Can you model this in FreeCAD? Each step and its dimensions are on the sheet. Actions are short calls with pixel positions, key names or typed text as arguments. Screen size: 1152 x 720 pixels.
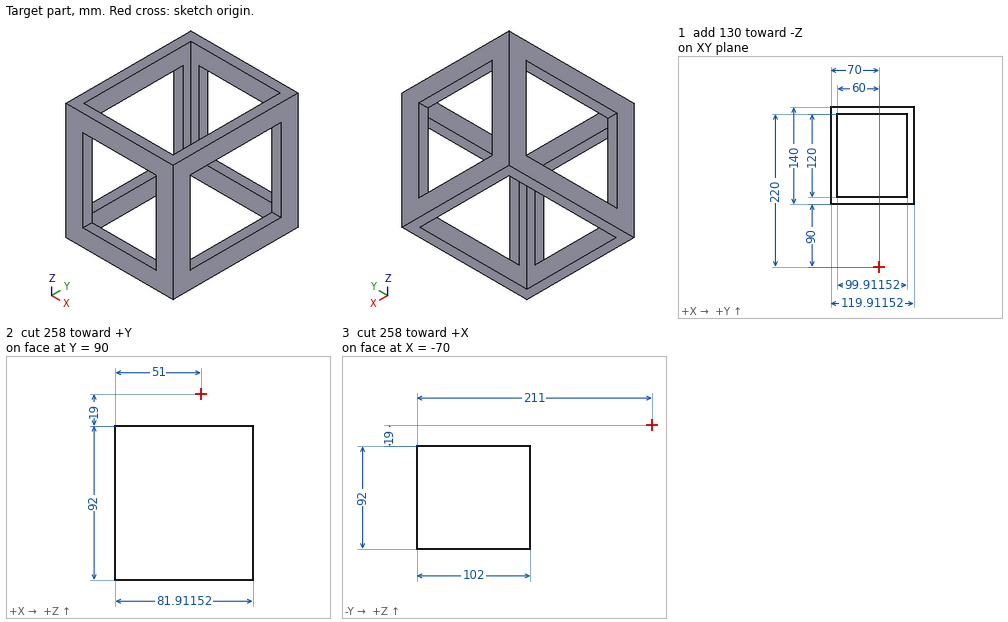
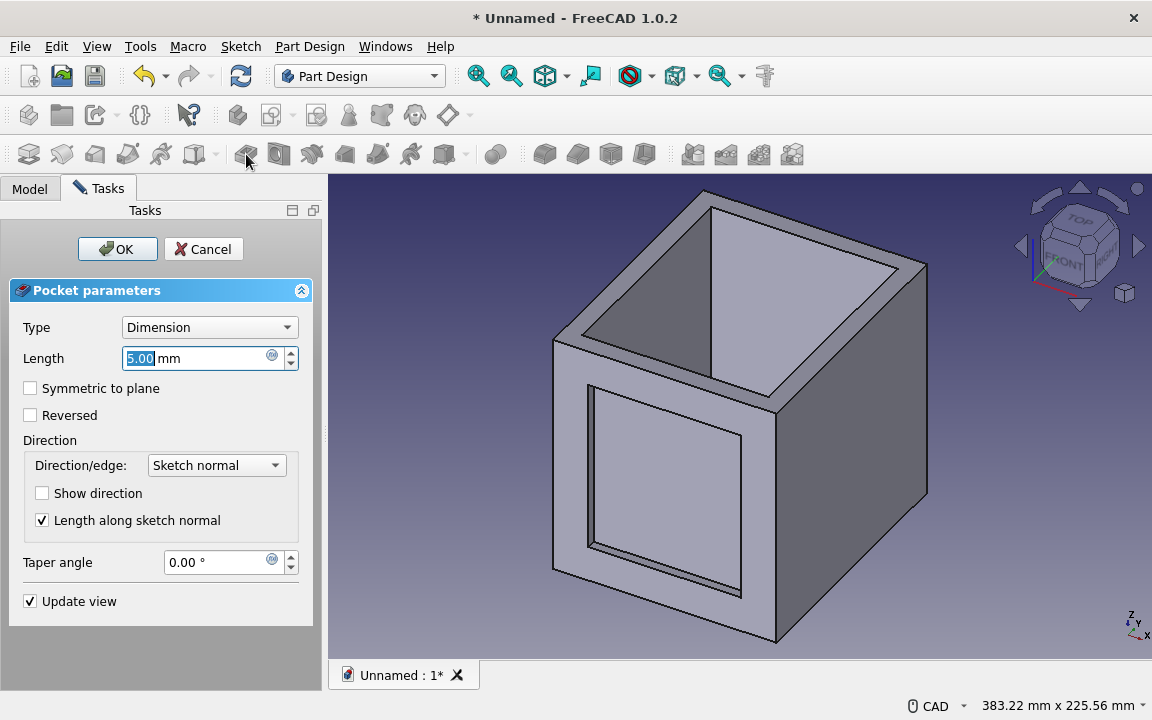
text(258)
key(Tab)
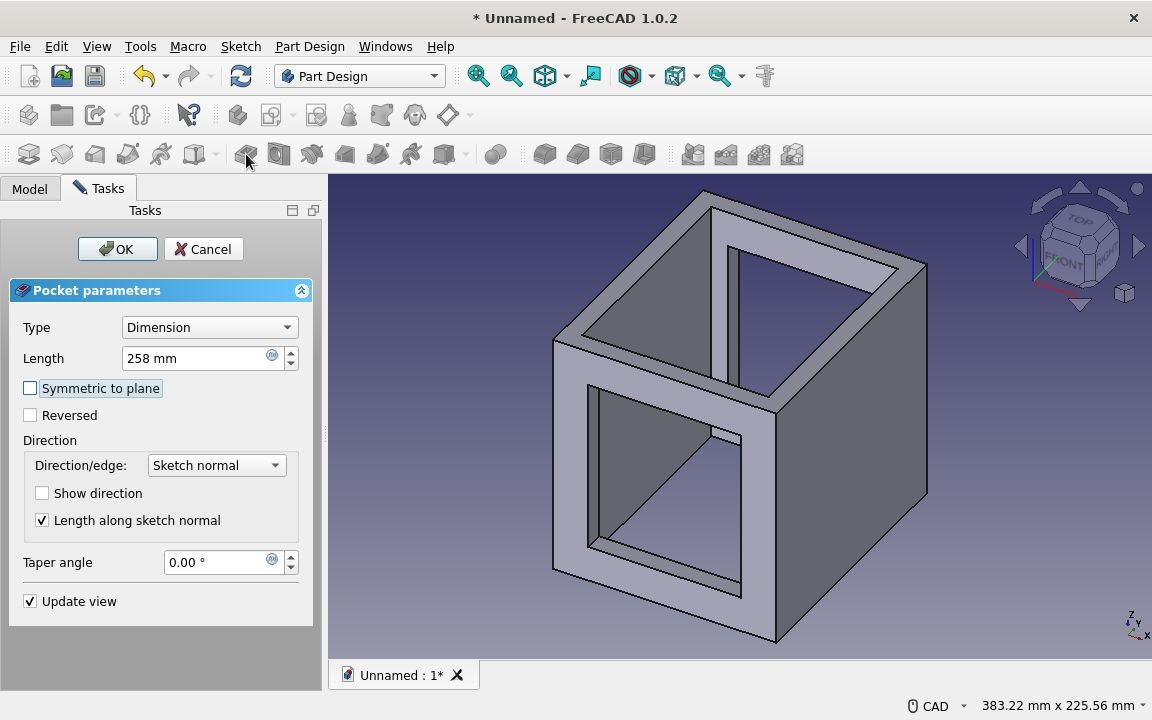
click(118, 249)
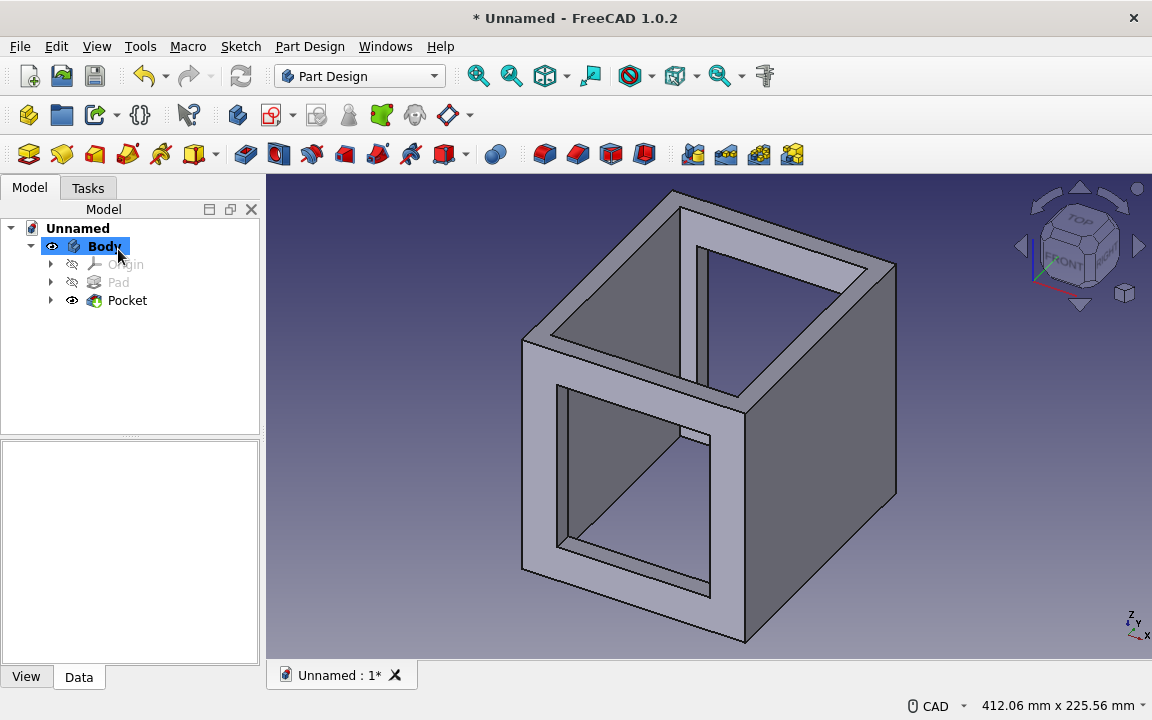
key(6)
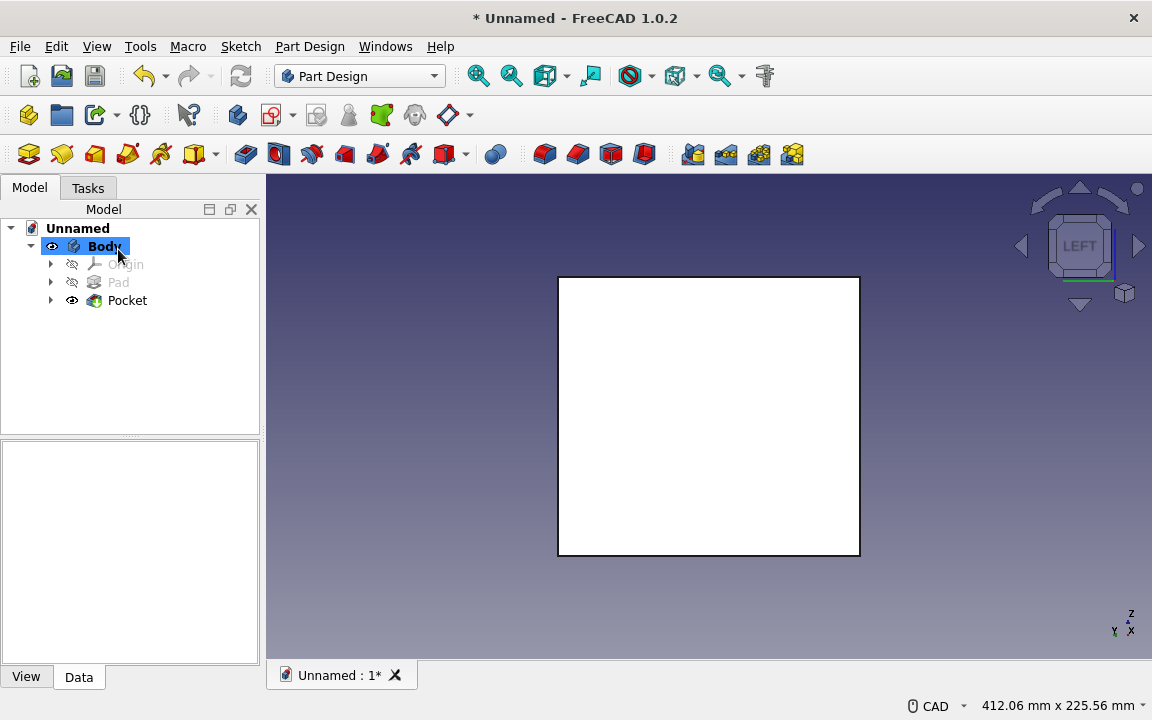
click(709, 415)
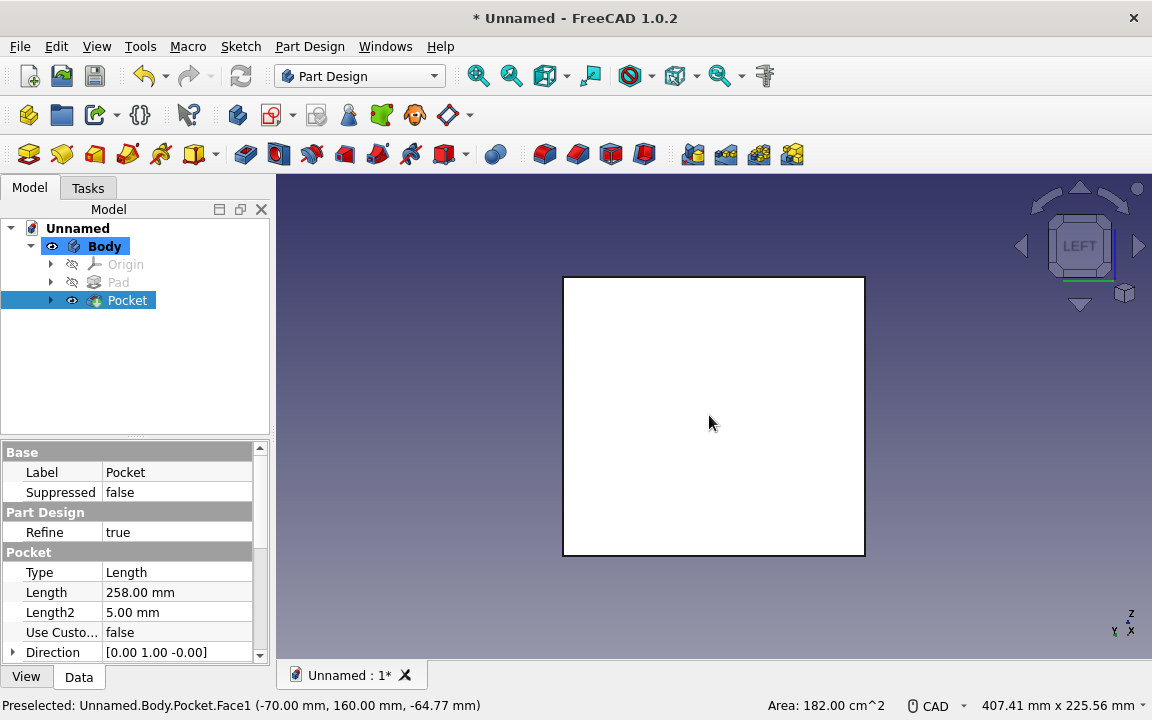
click(270, 116)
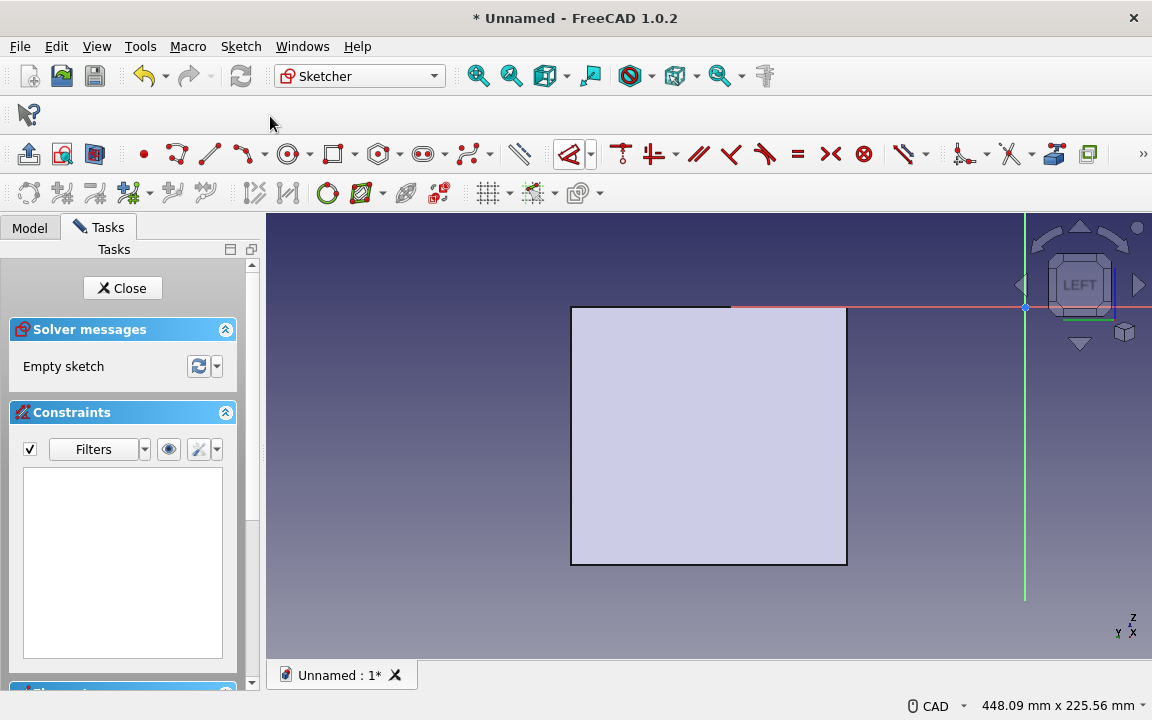
scroll(294, 521, down, 1)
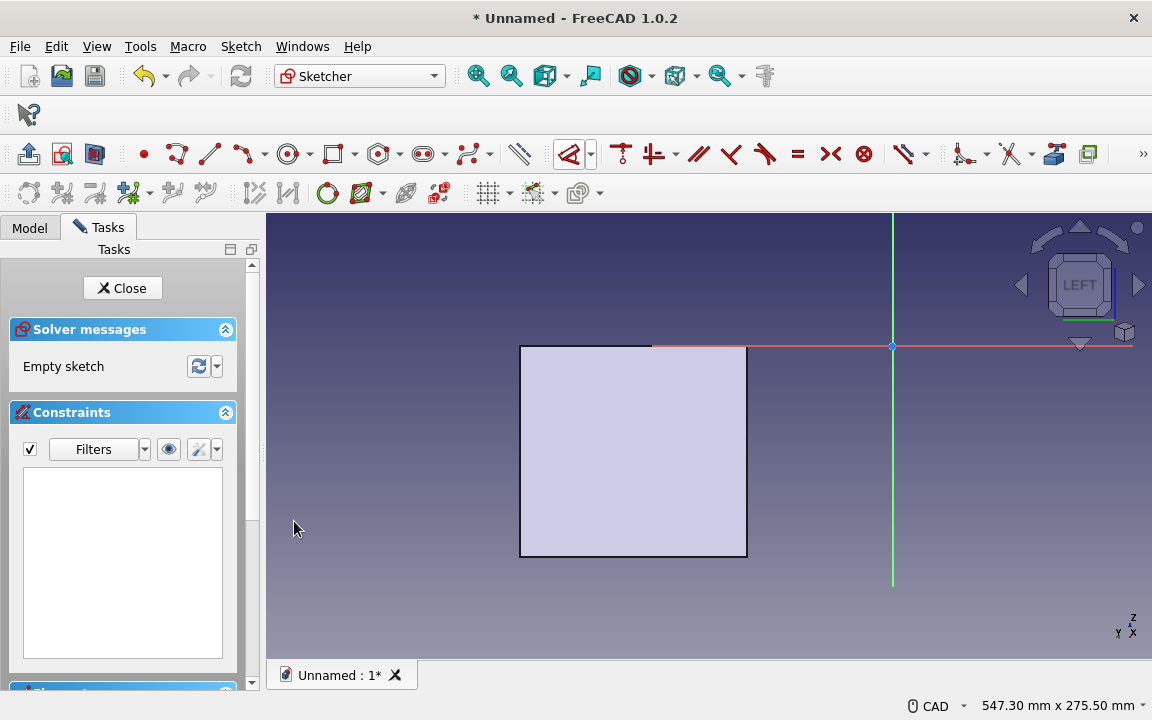
scroll(888, 436, up, 2)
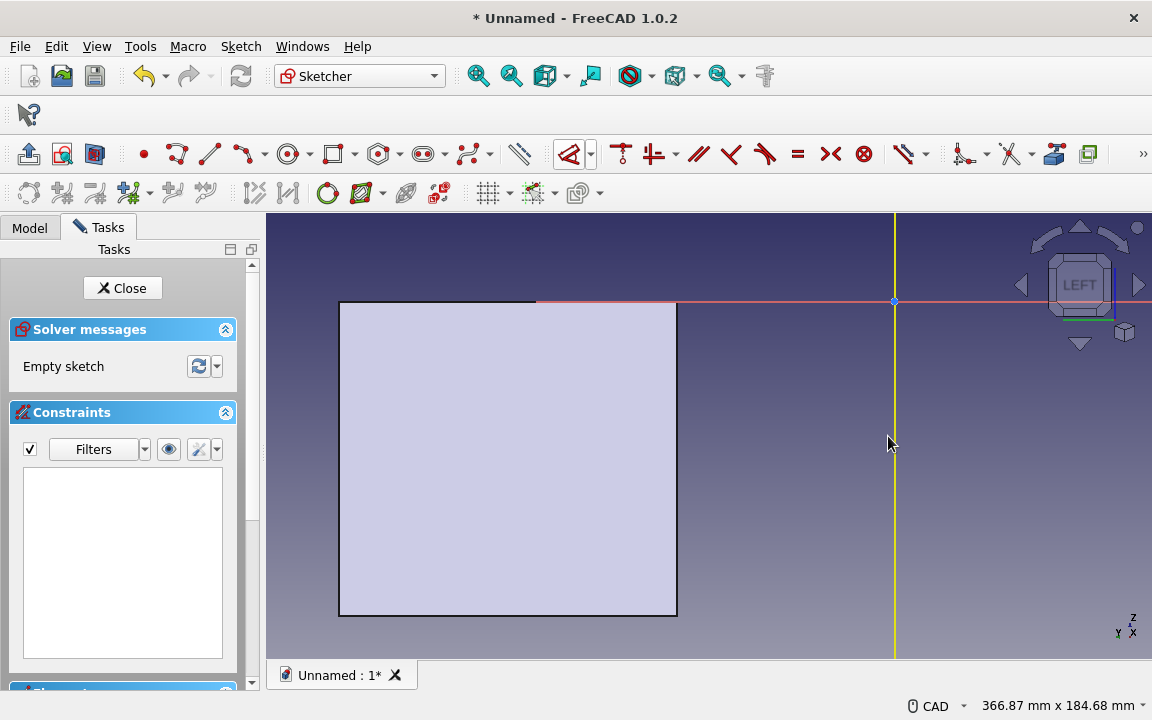
click(332, 154)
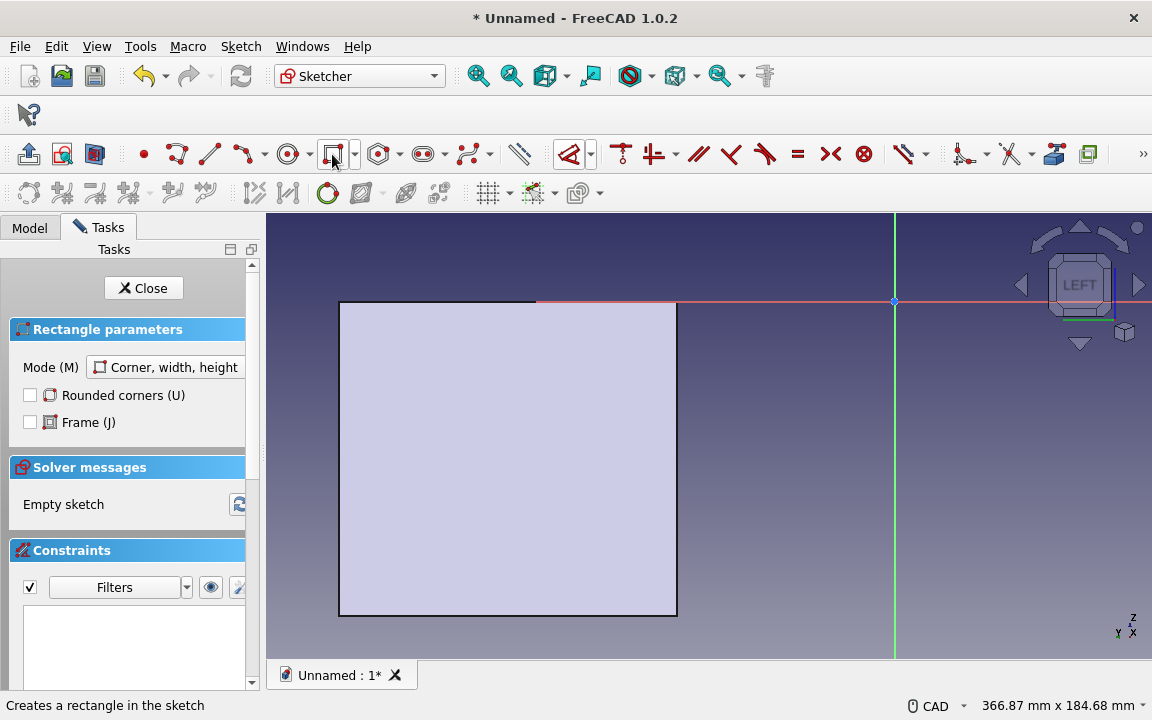
click(385, 348)
click(632, 570)
key(Escape)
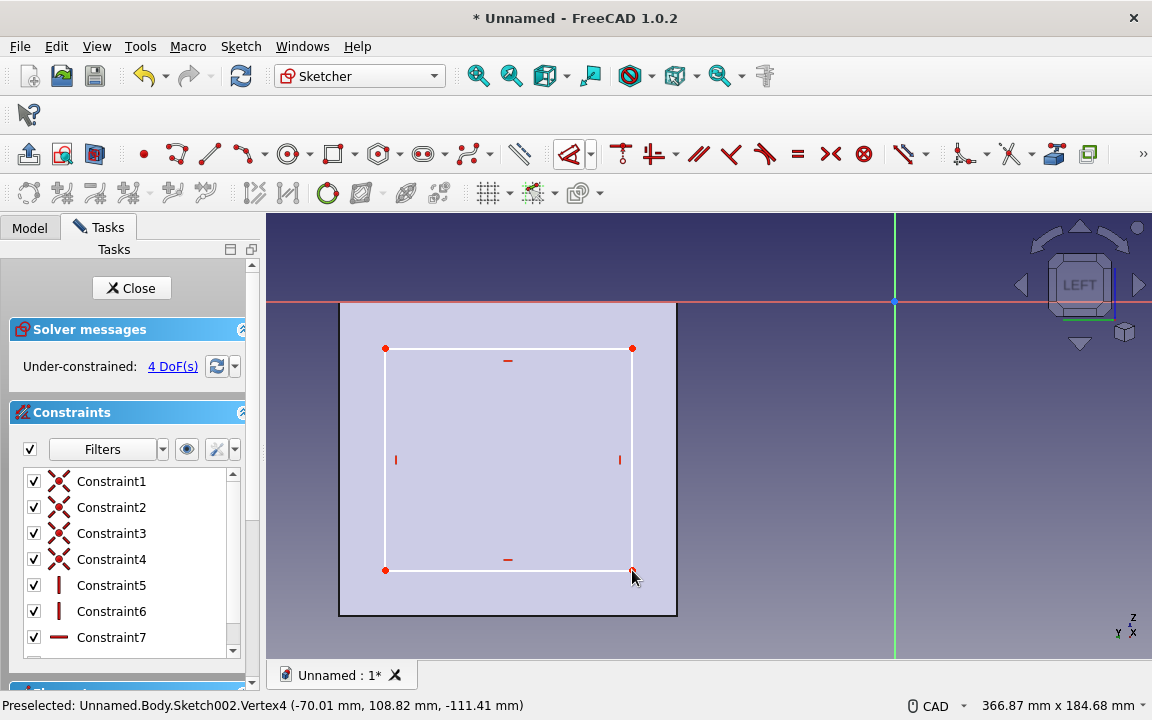
click(385, 416)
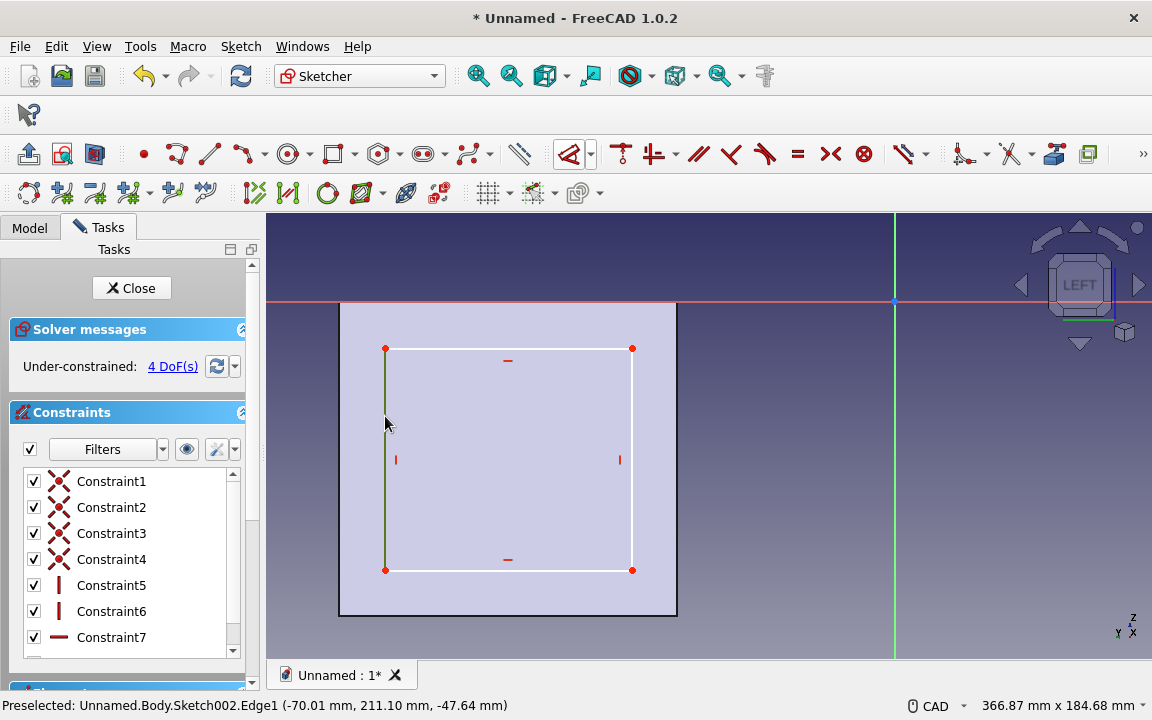
key(i)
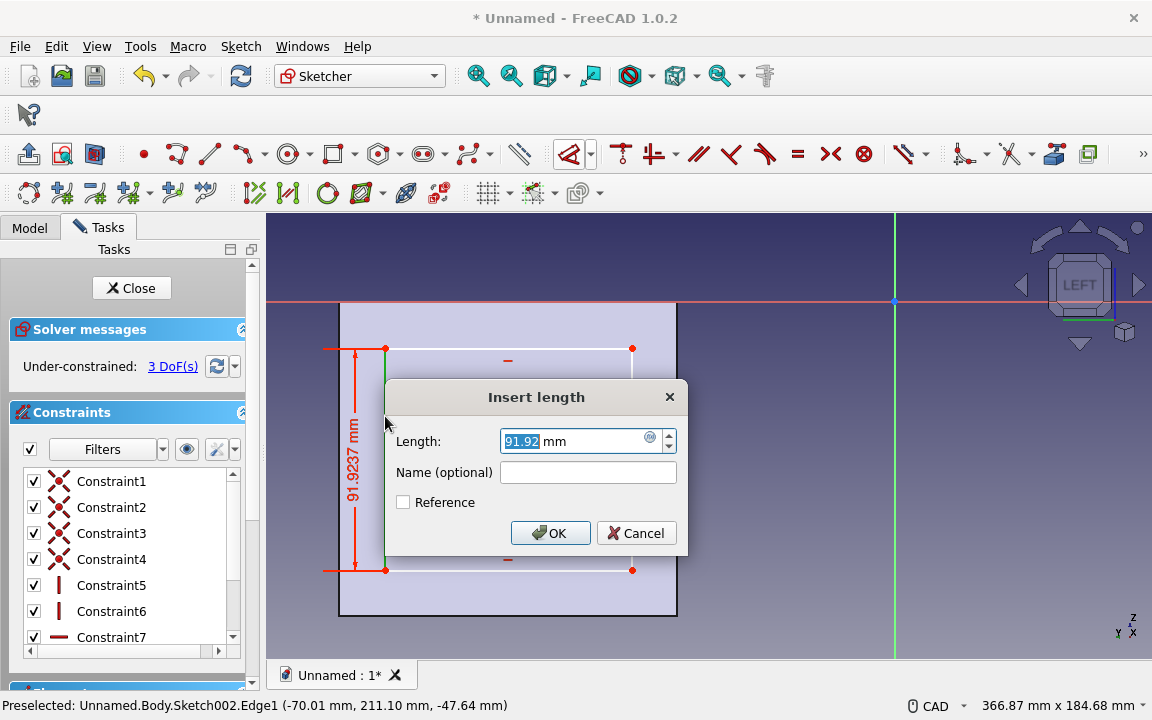
text(92)
key(Return)